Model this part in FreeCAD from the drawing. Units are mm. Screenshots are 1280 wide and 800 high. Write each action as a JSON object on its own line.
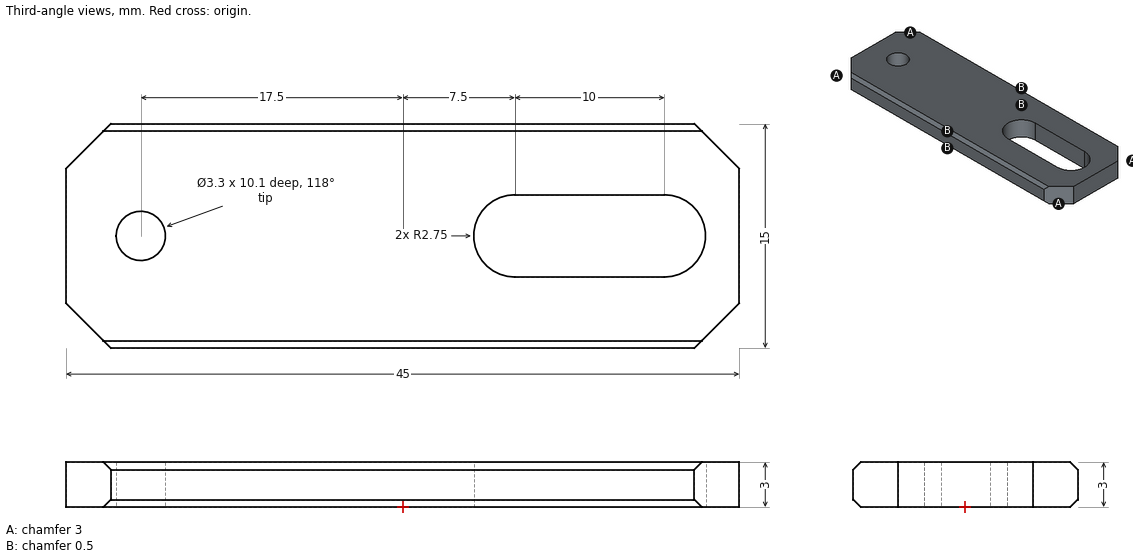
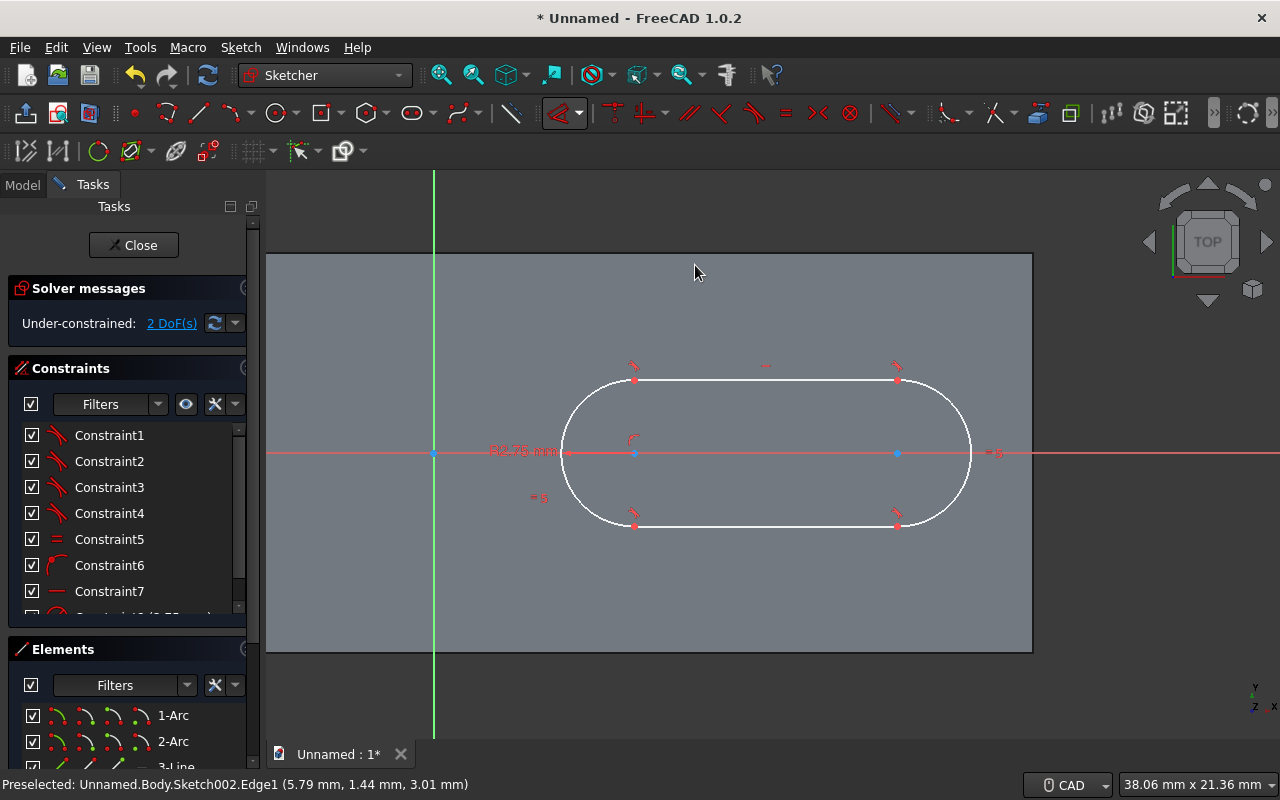
{"action": "left_click", "coordinate": [714, 380]}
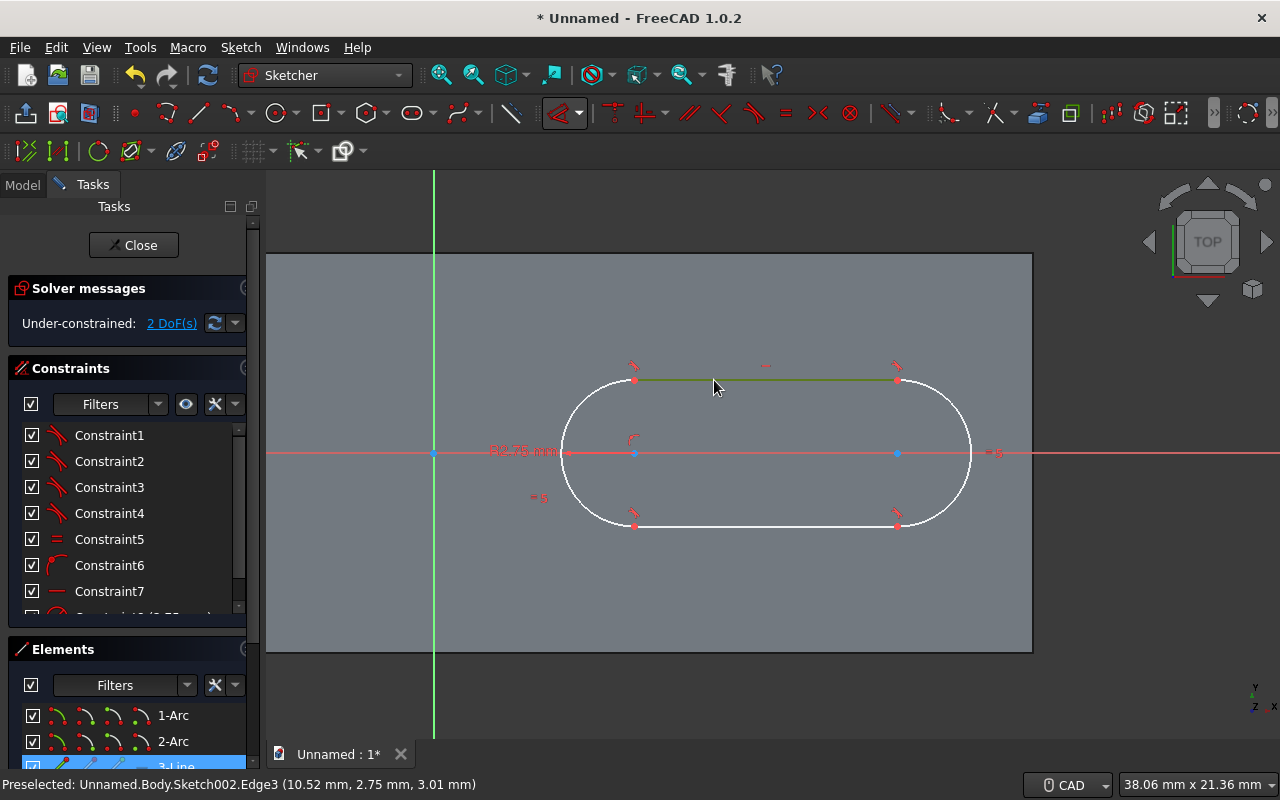
{"action": "left_click", "coordinate": [582, 114]}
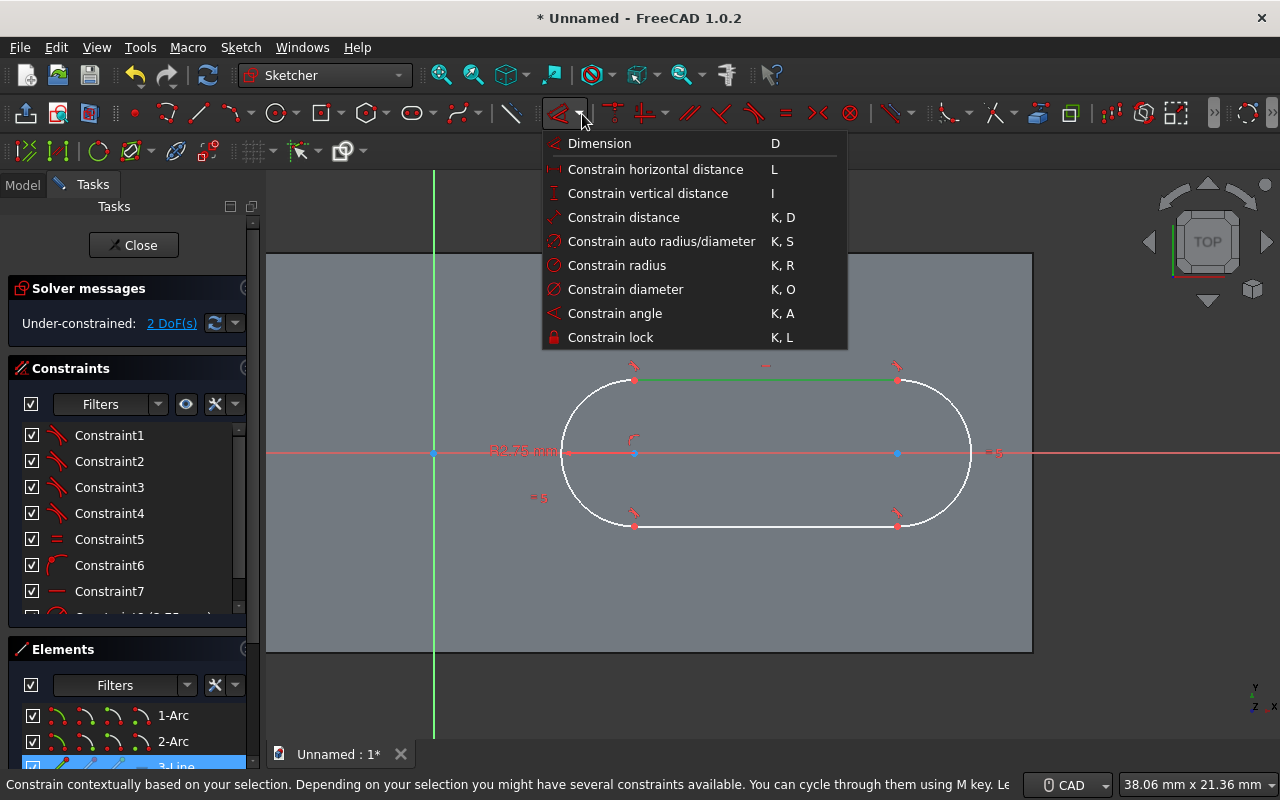
{"action": "left_click", "coordinate": [695, 169]}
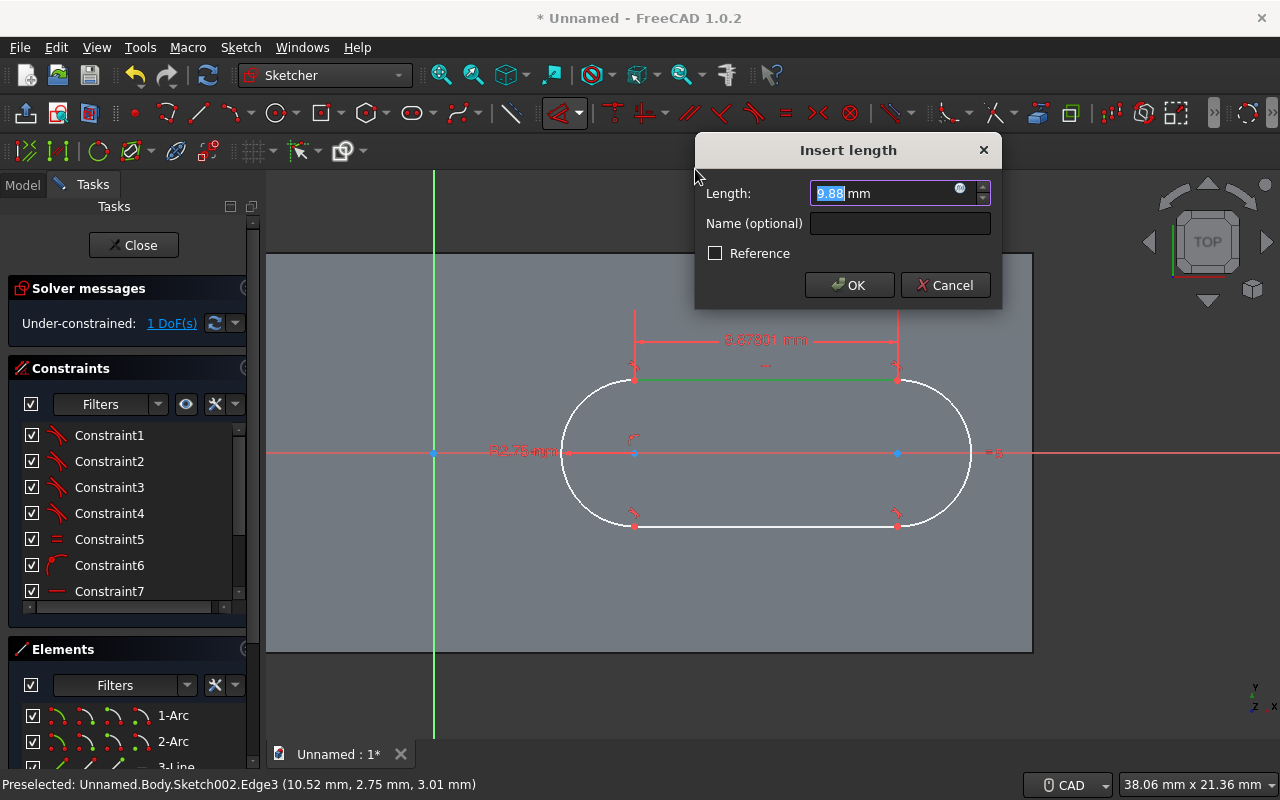
{"action": "type", "text": "10"}
{"action": "key", "text": "Return"}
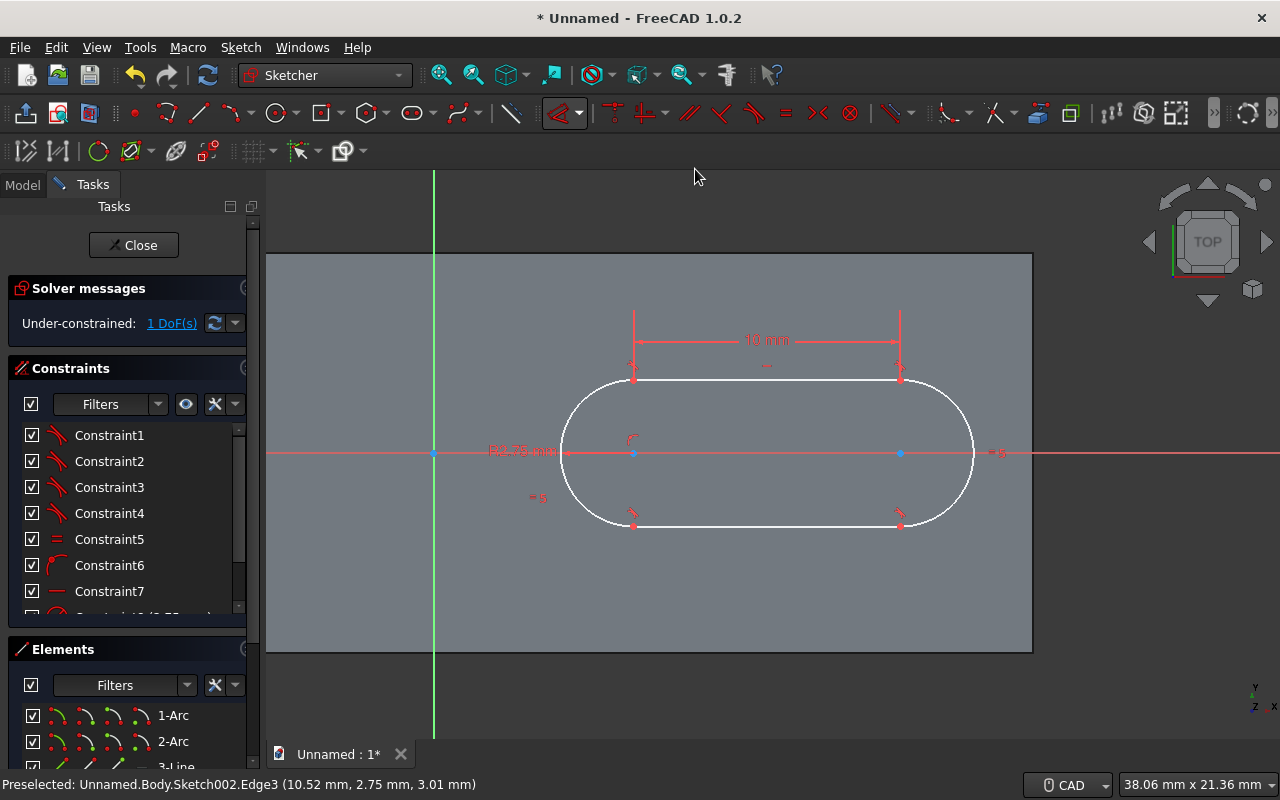
{"action": "left_click", "coordinate": [634, 380]}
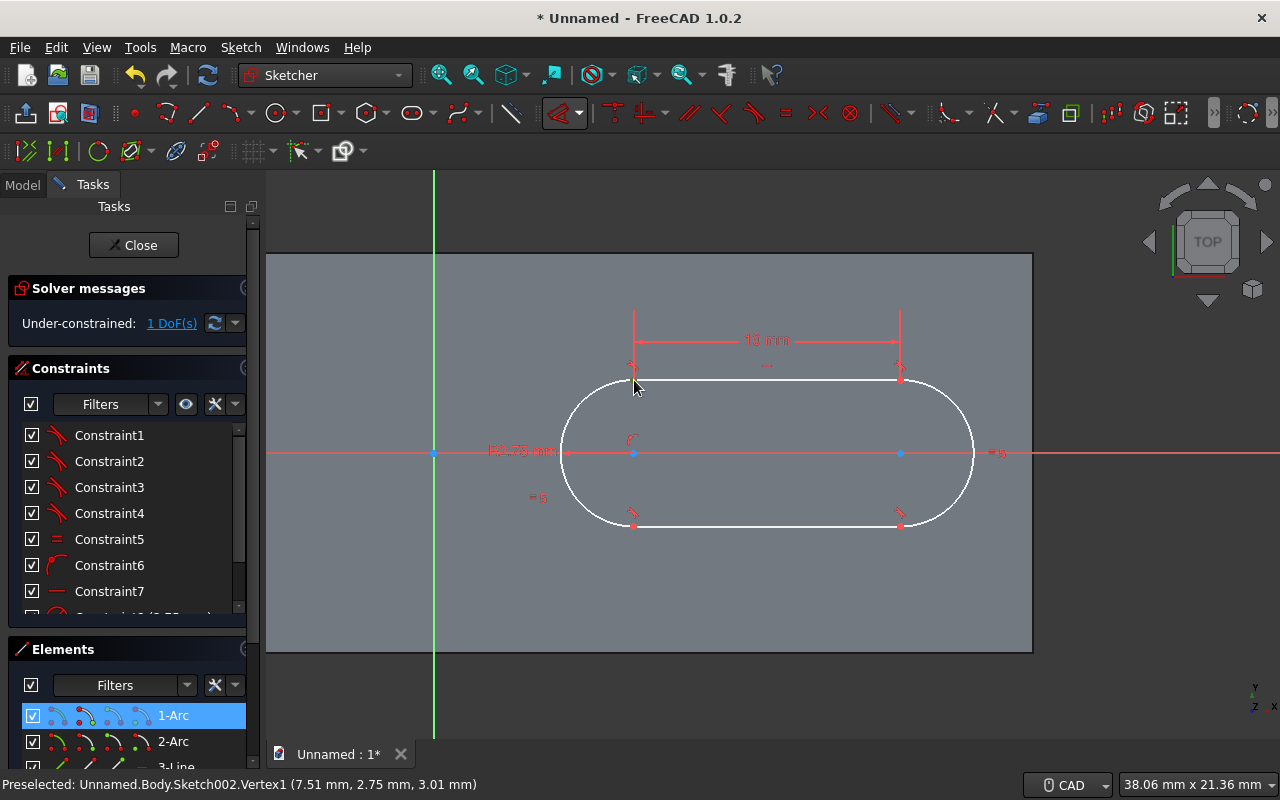
{"action": "left_click", "coordinate": [582, 114]}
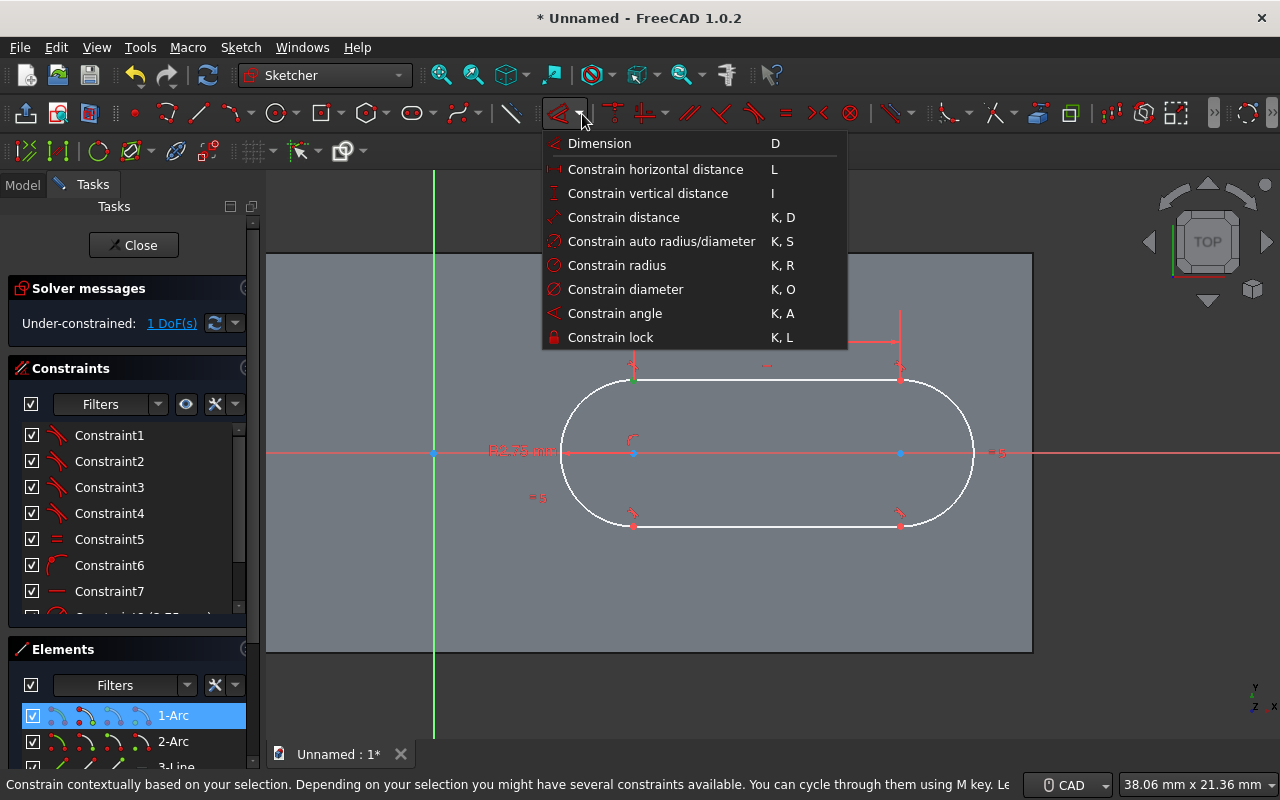
{"action": "left_click", "coordinate": [695, 169]}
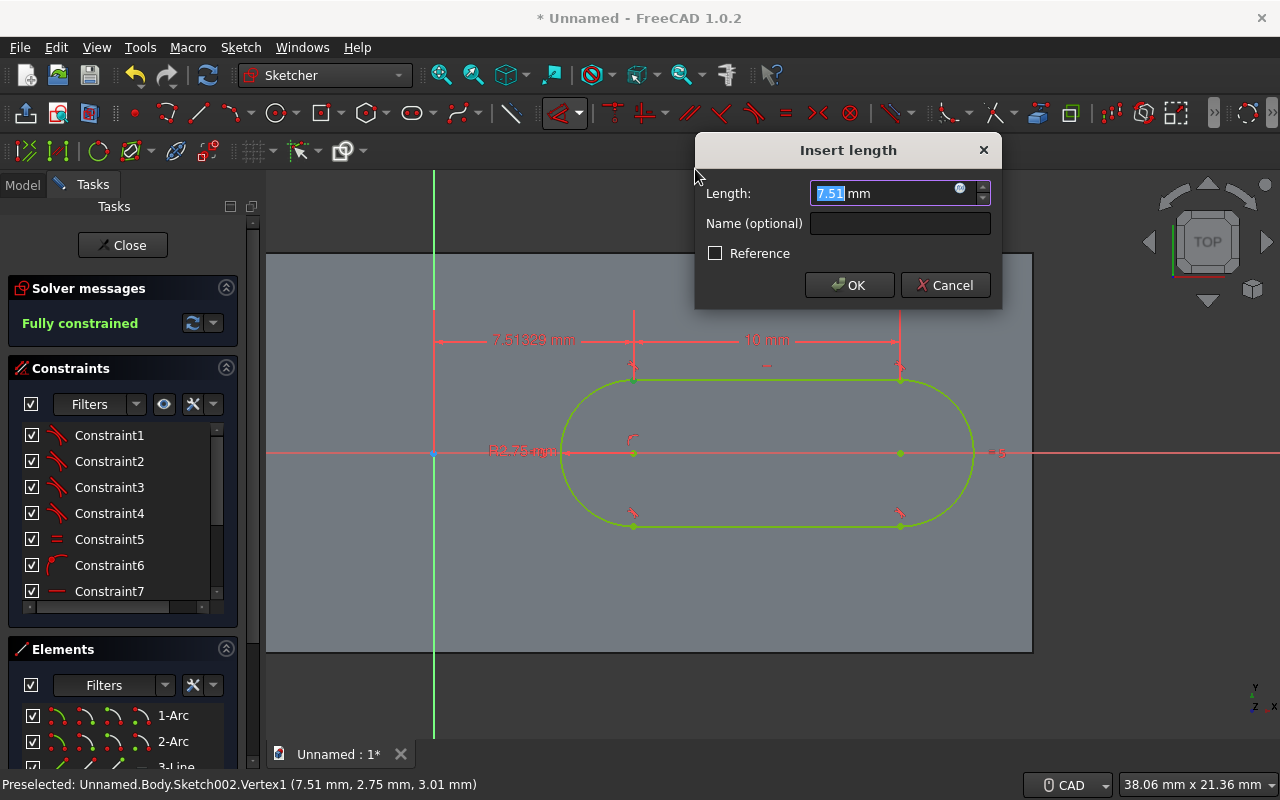
{"action": "type", "text": "7.5"}
{"action": "key", "text": "Return"}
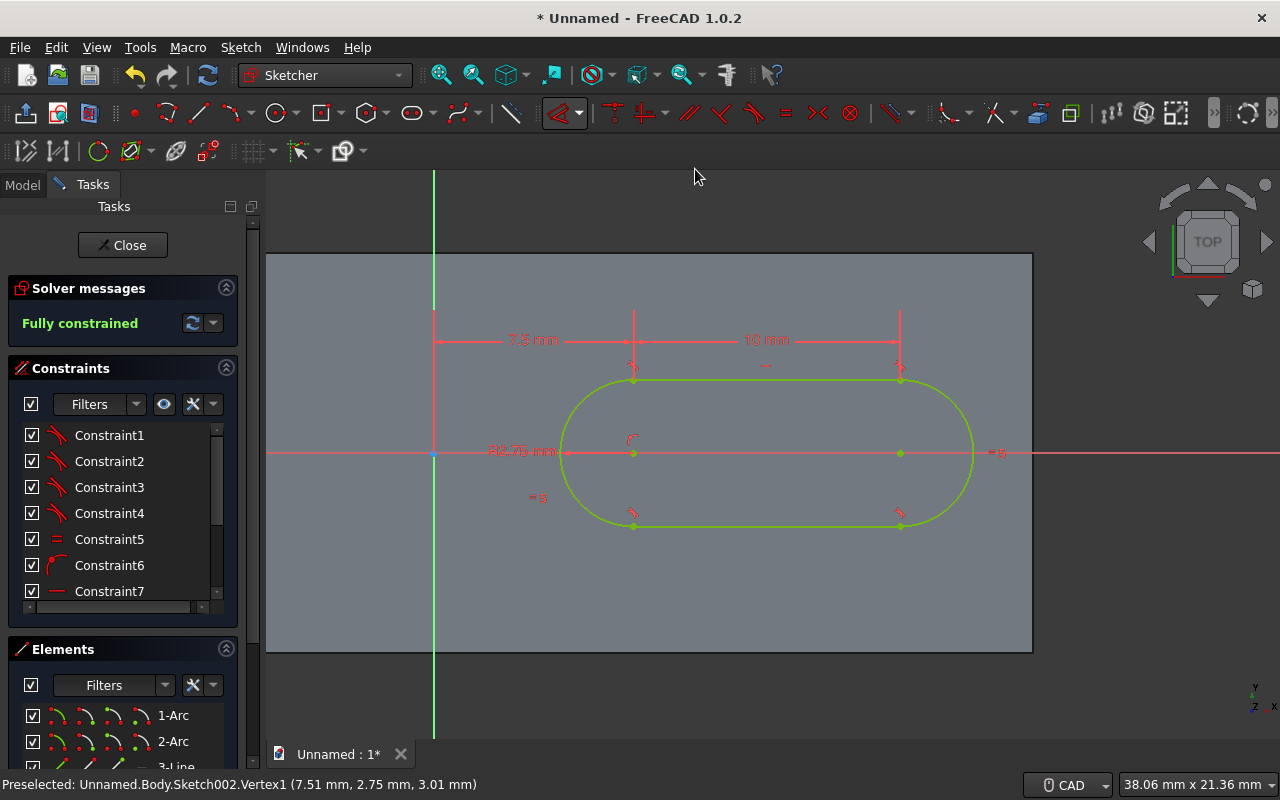
{"action": "left_click", "coordinate": [123, 245]}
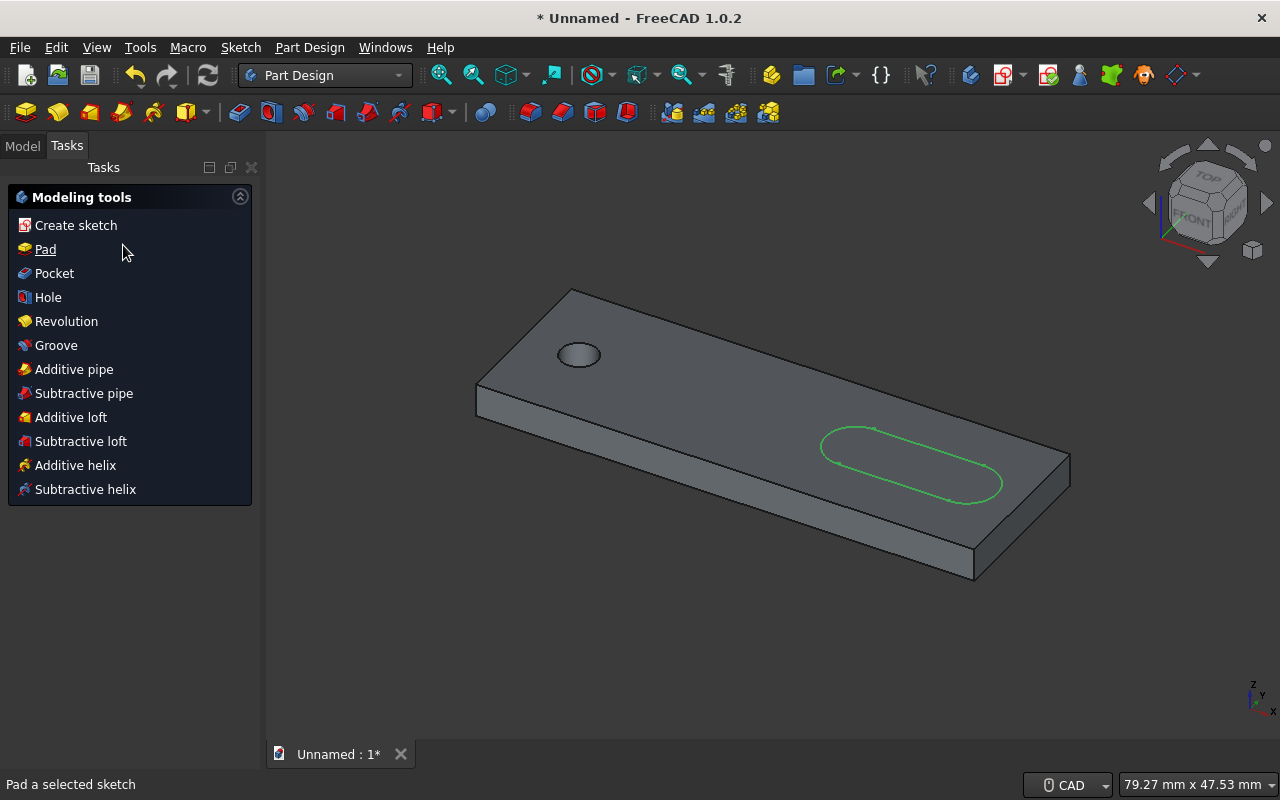
{"action": "left_click", "coordinate": [240, 112]}